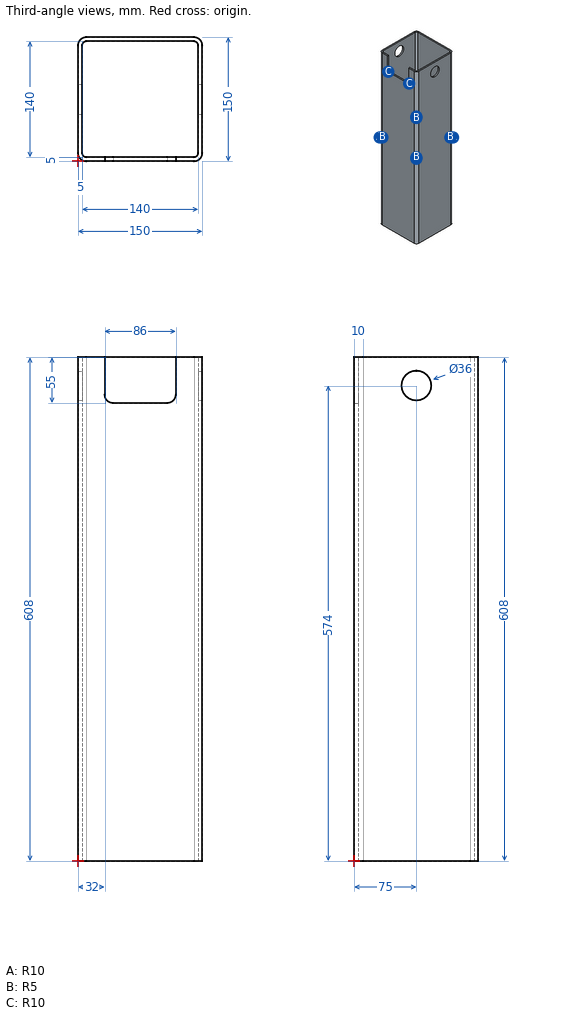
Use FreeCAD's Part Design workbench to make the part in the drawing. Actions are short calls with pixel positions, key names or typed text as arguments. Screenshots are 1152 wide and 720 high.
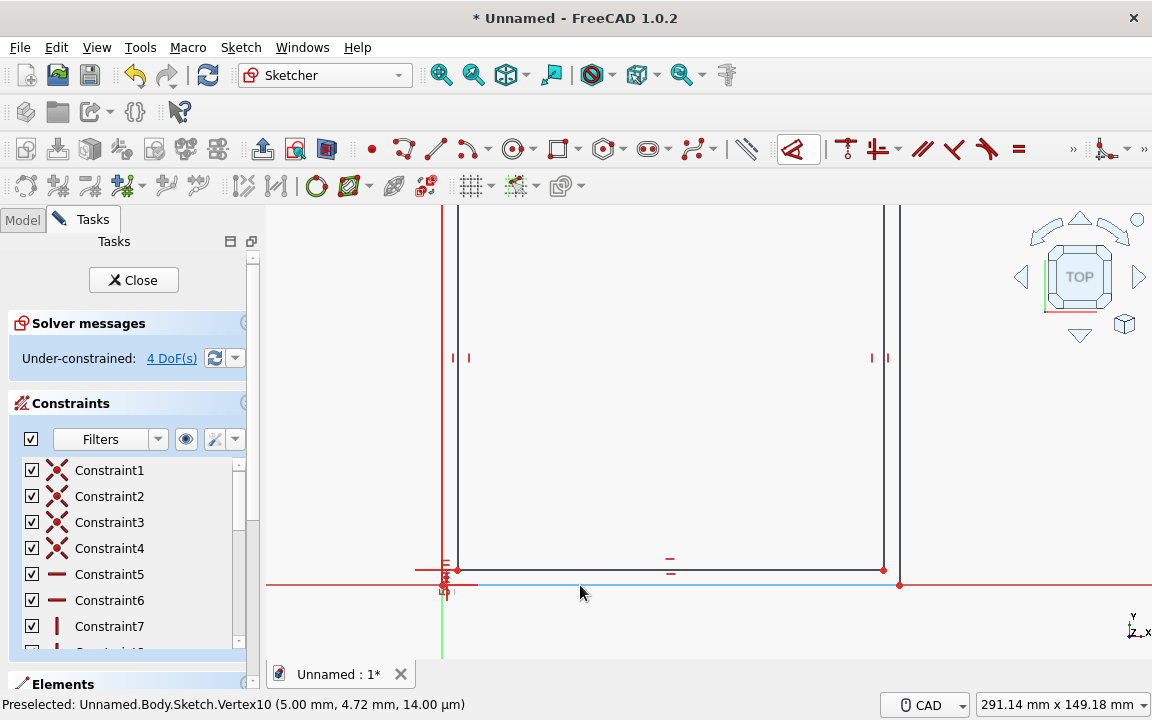
click(580, 585)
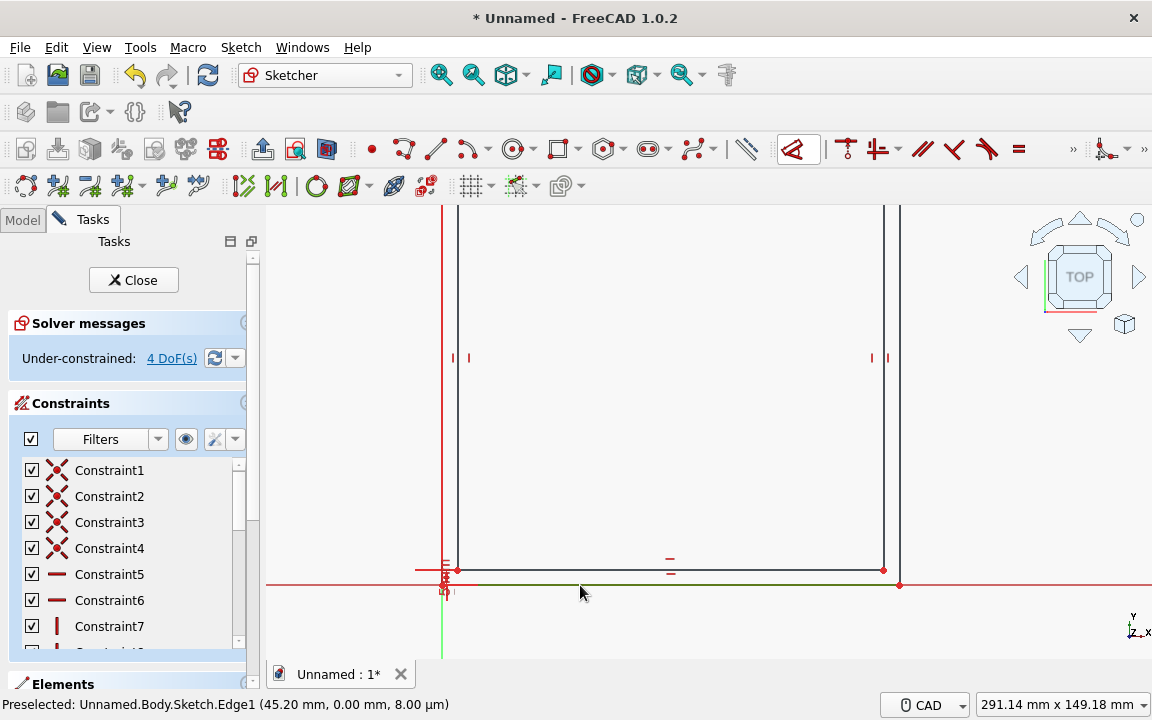
key(l)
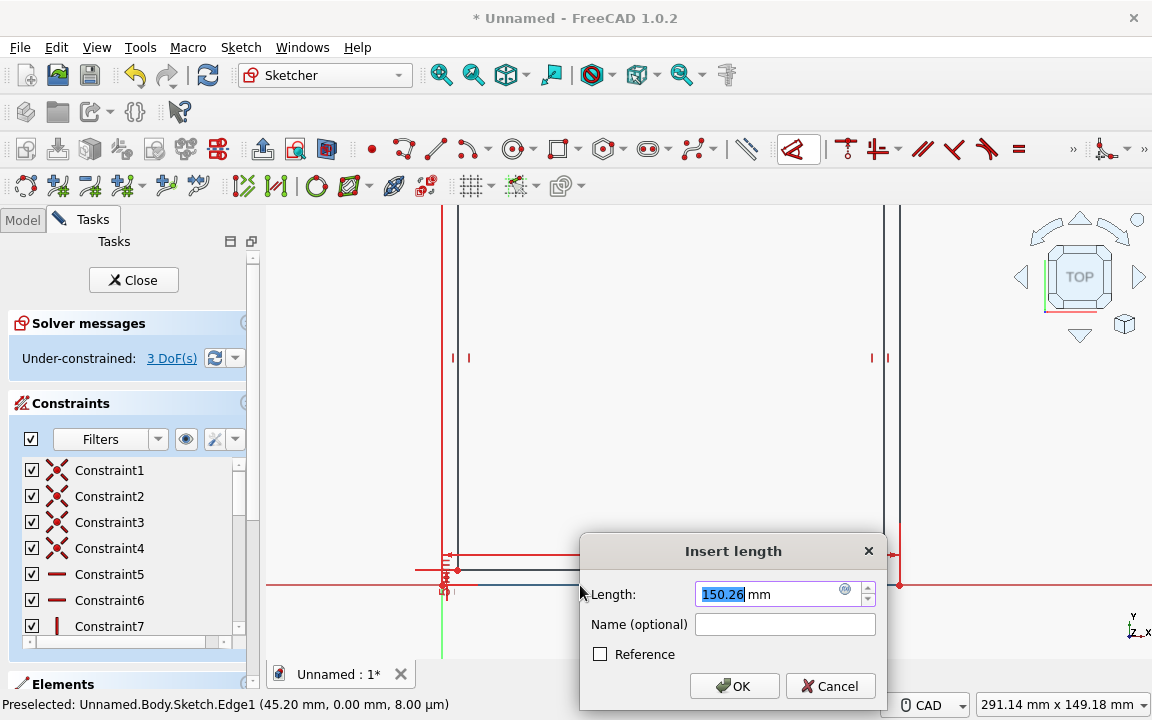
text(150)
key(Return)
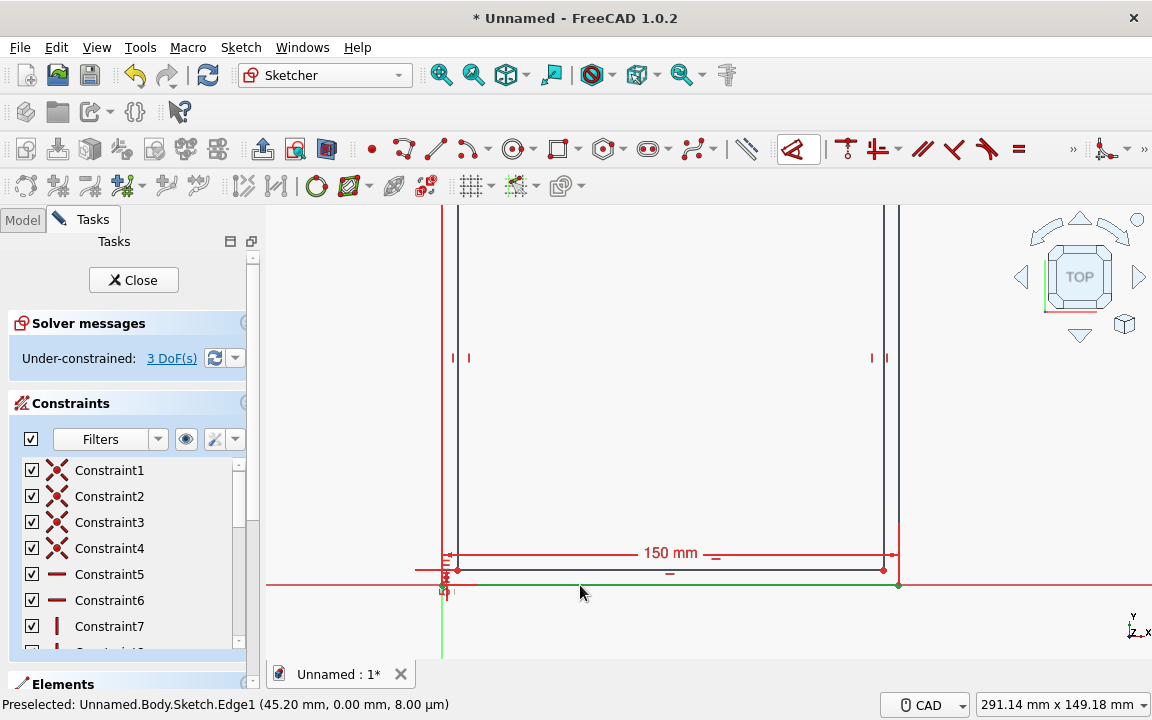
click(899, 449)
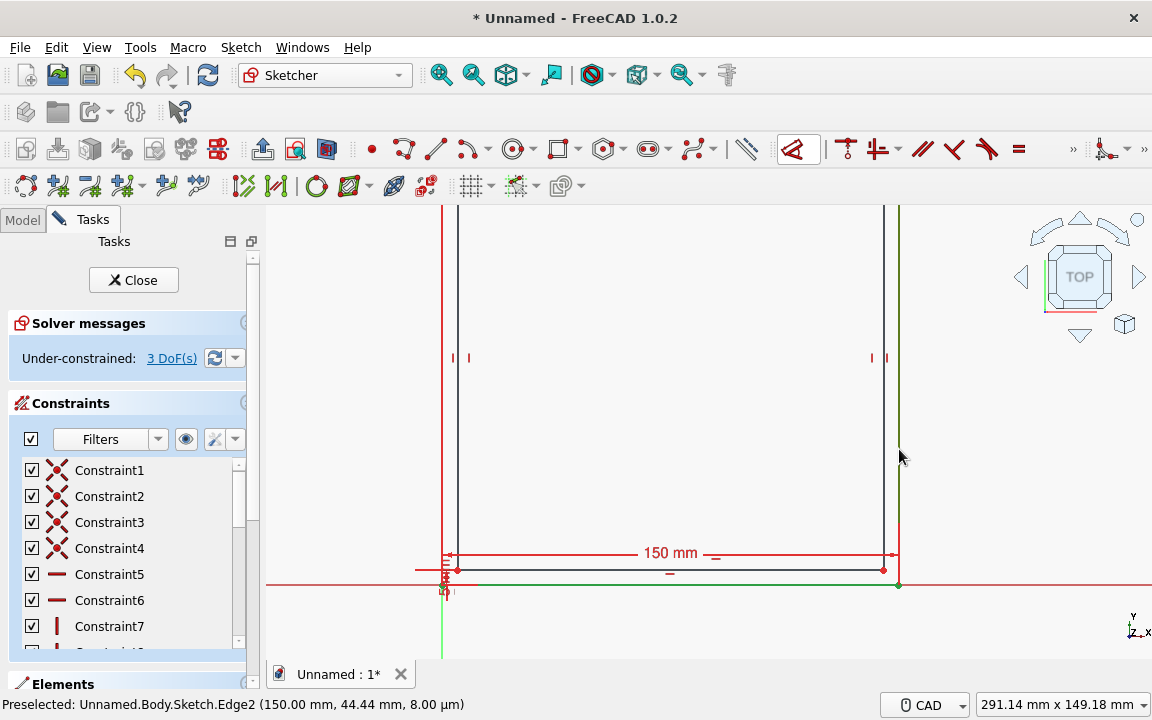
key(i)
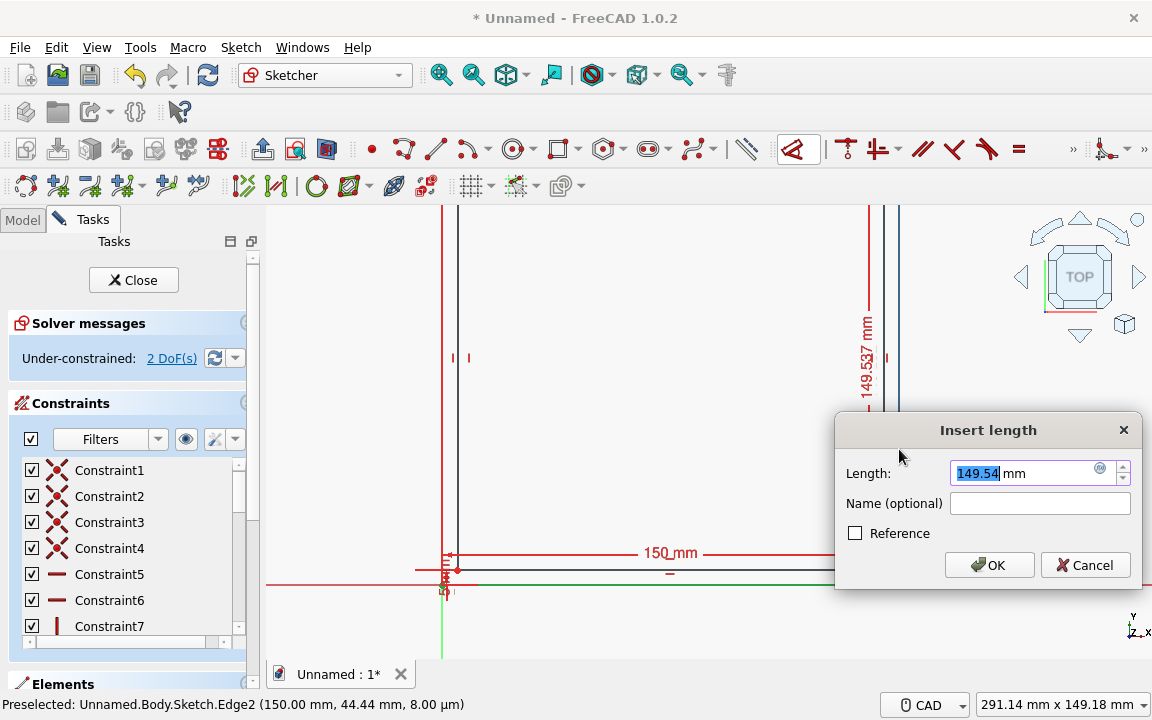
text(150)
key(Return)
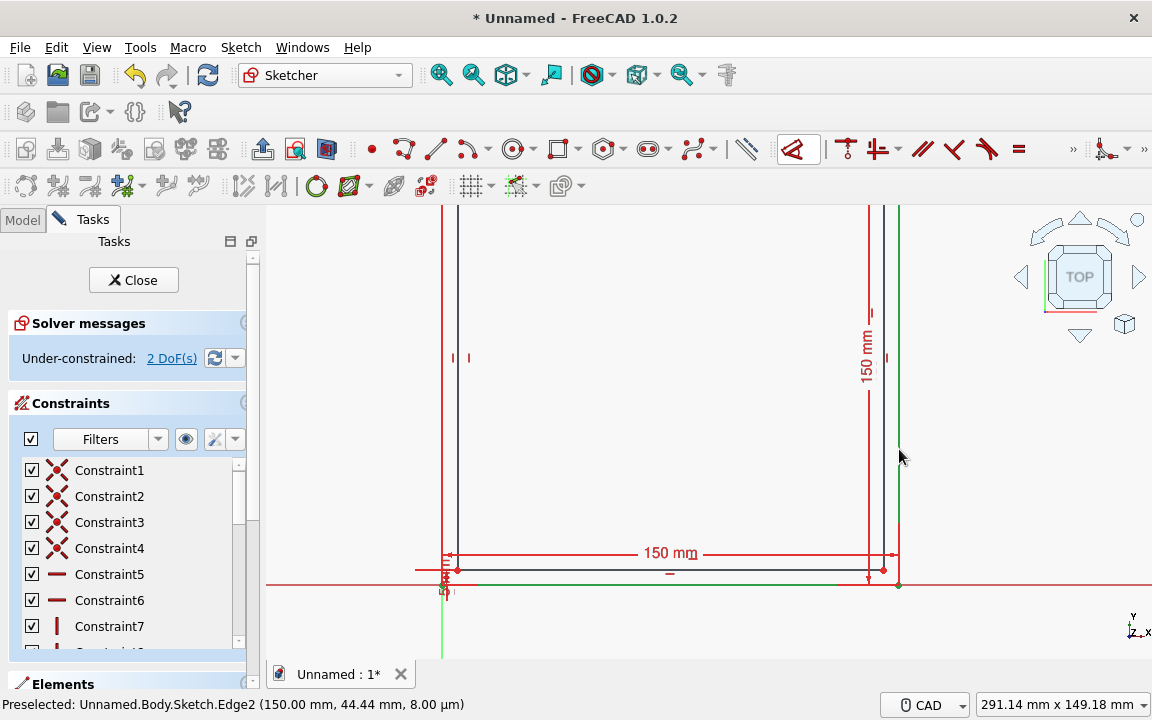
click(458, 273)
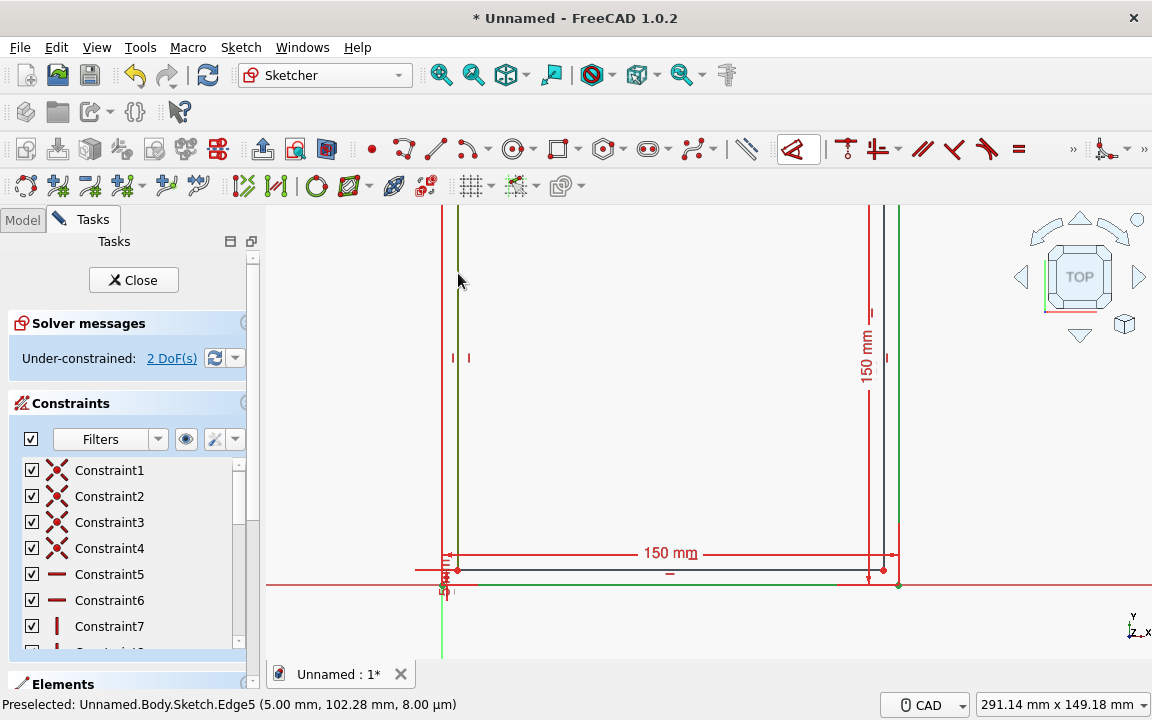
key(i)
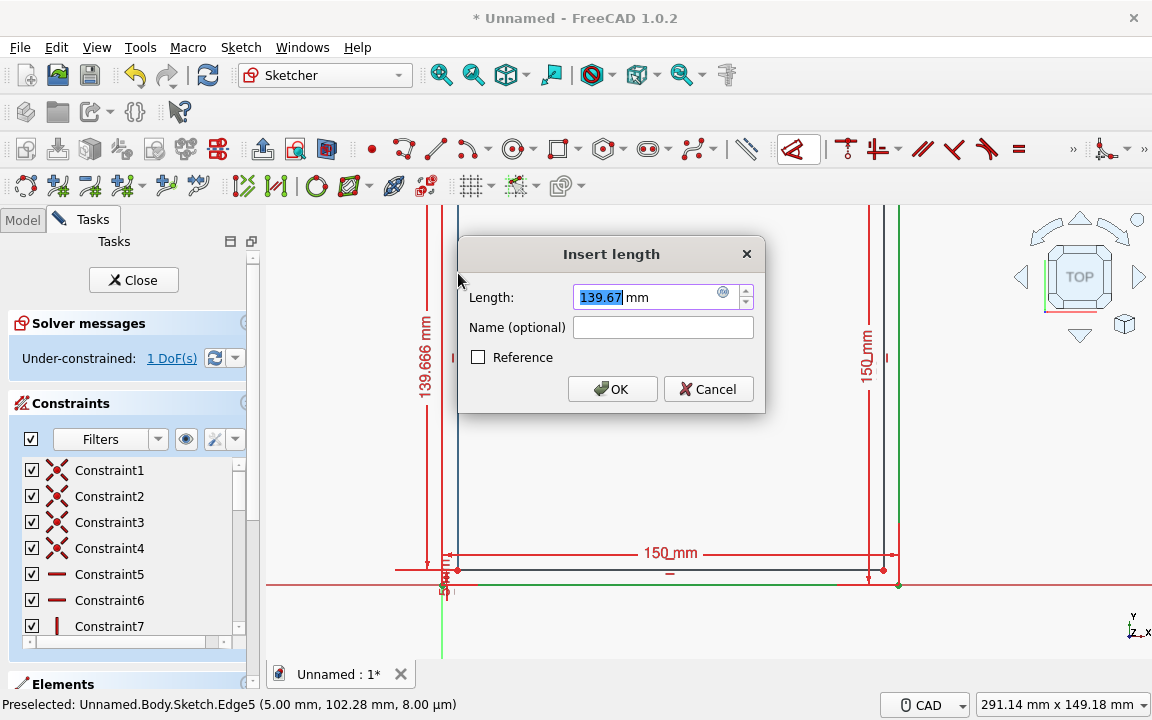
text(140)
key(Return)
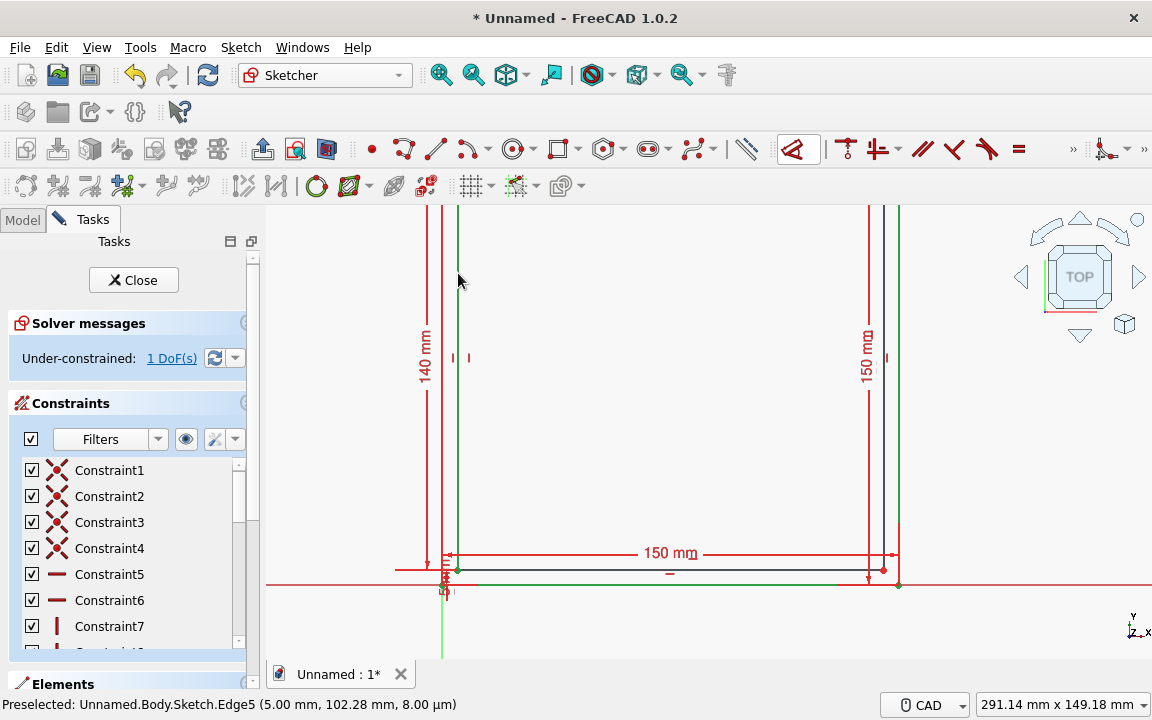
click(585, 570)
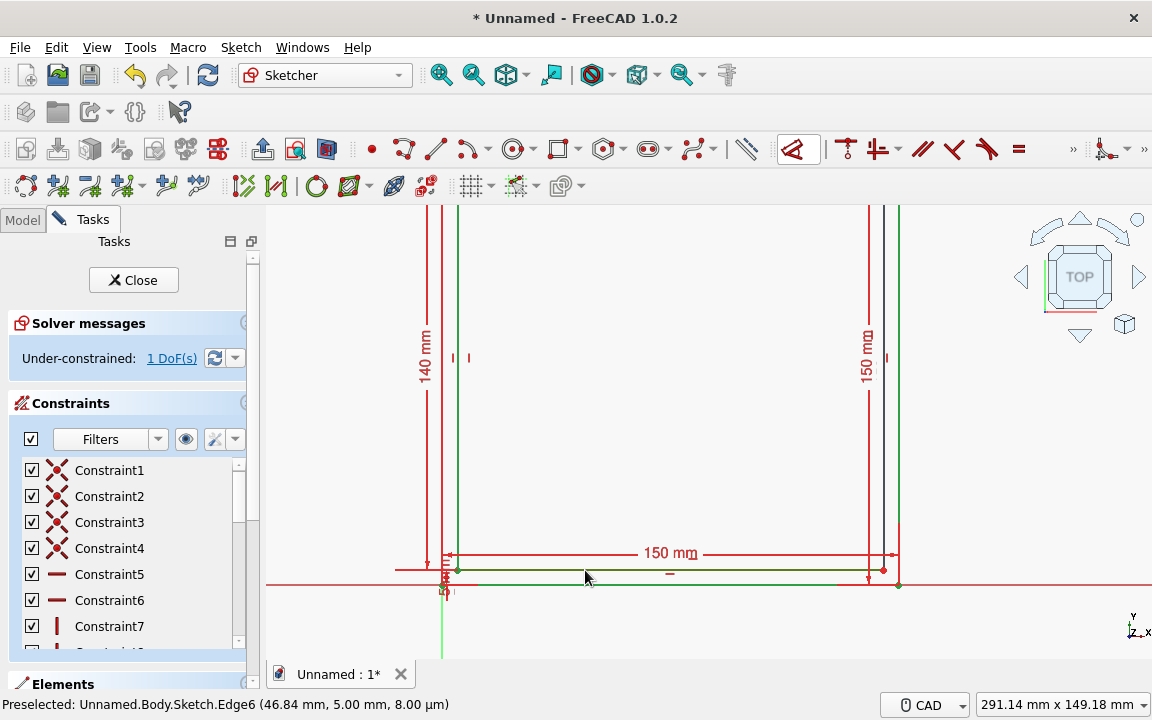
click(814, 150)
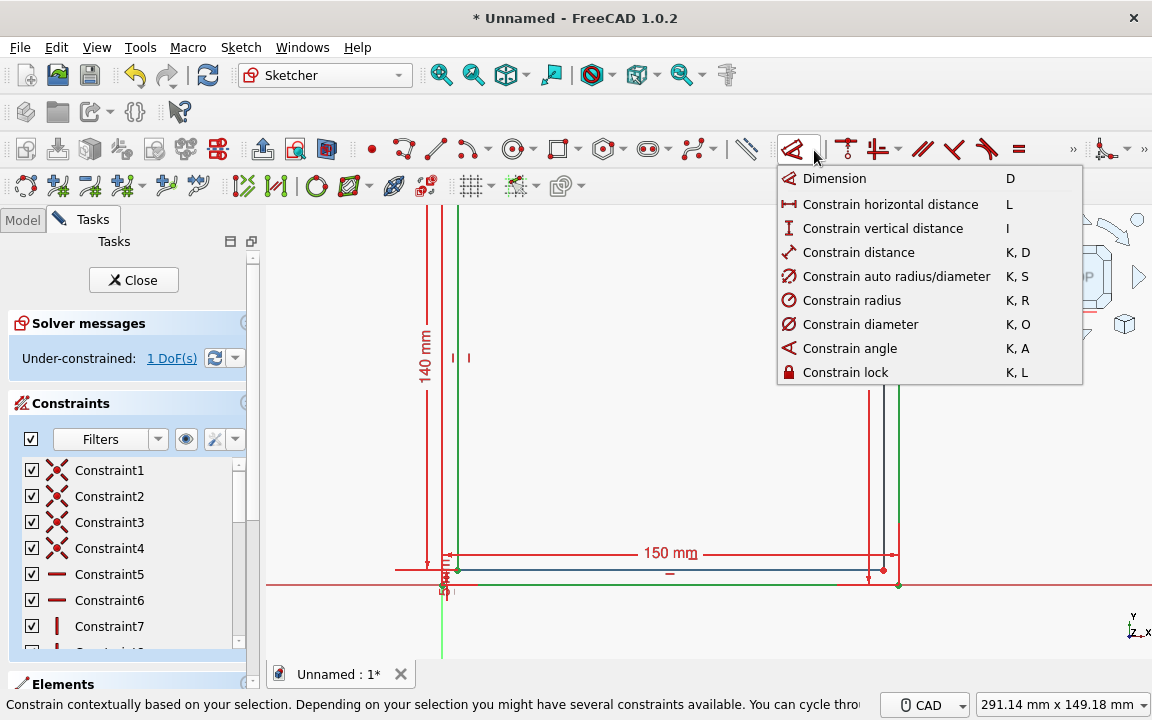
click(930, 204)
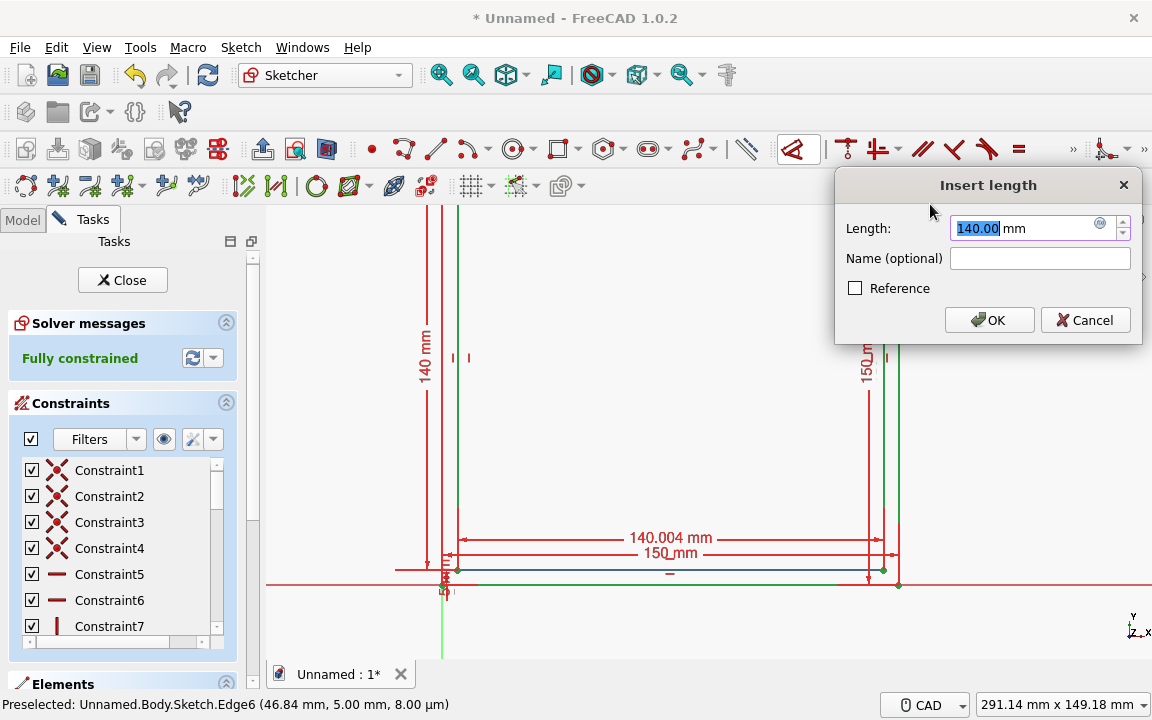
text(140)
key(Return)